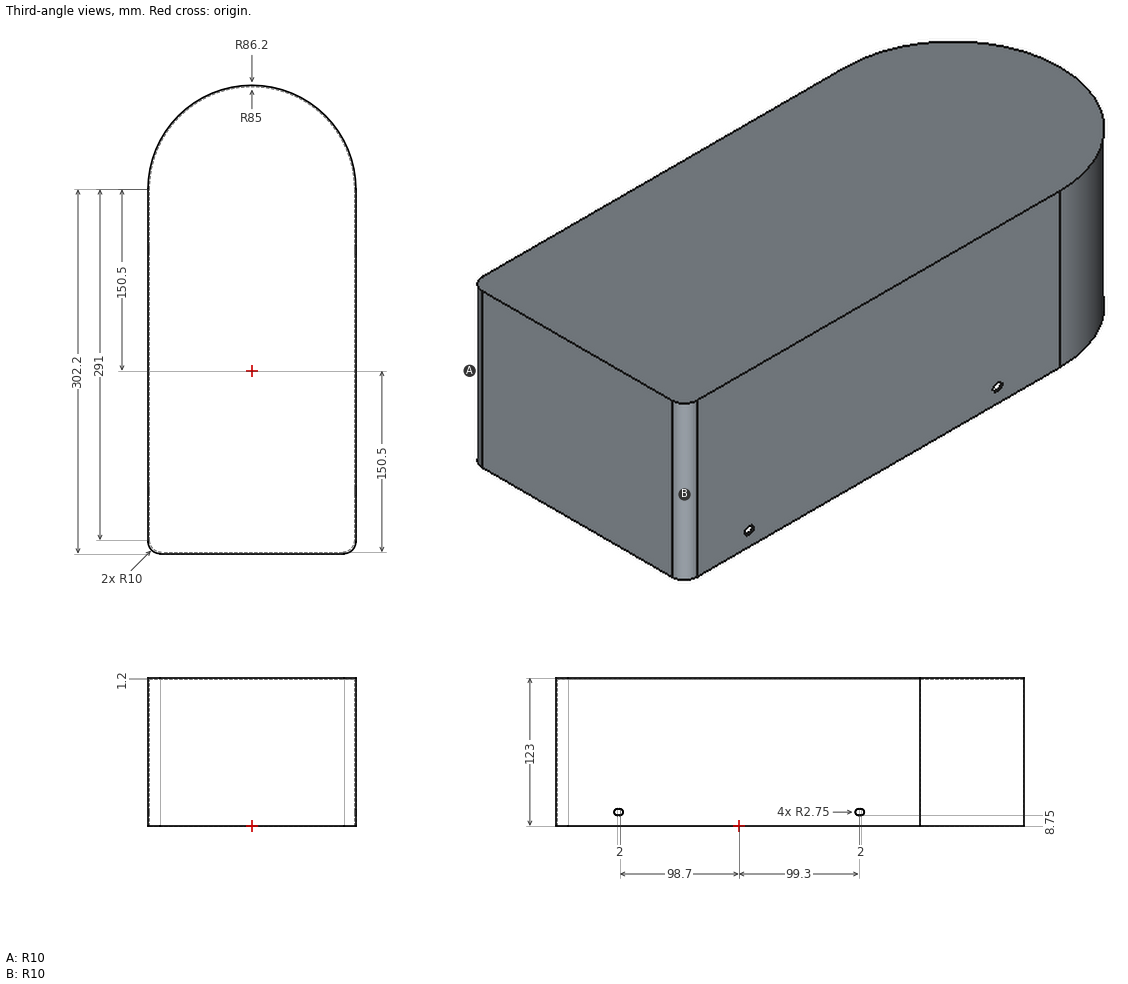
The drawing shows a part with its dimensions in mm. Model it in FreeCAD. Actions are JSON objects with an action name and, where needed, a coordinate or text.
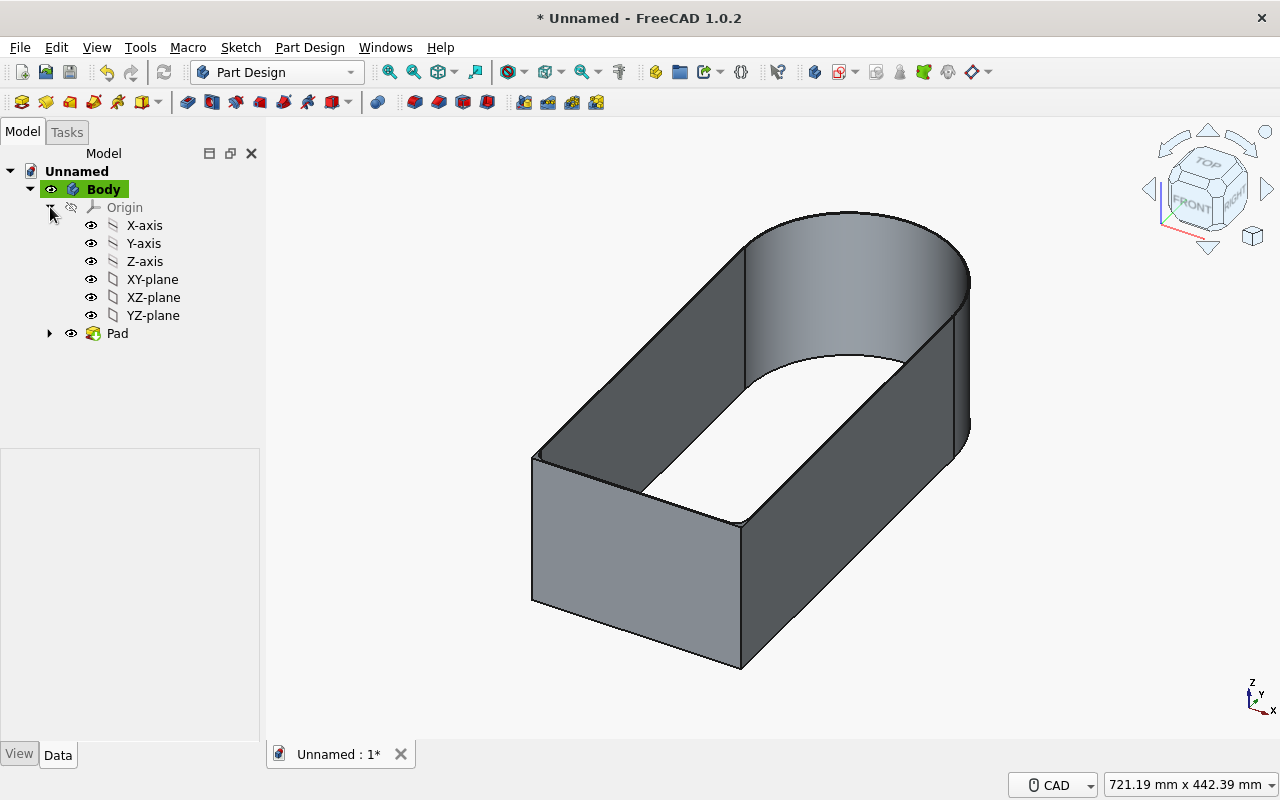
{"action": "left_click", "coordinate": [136, 279]}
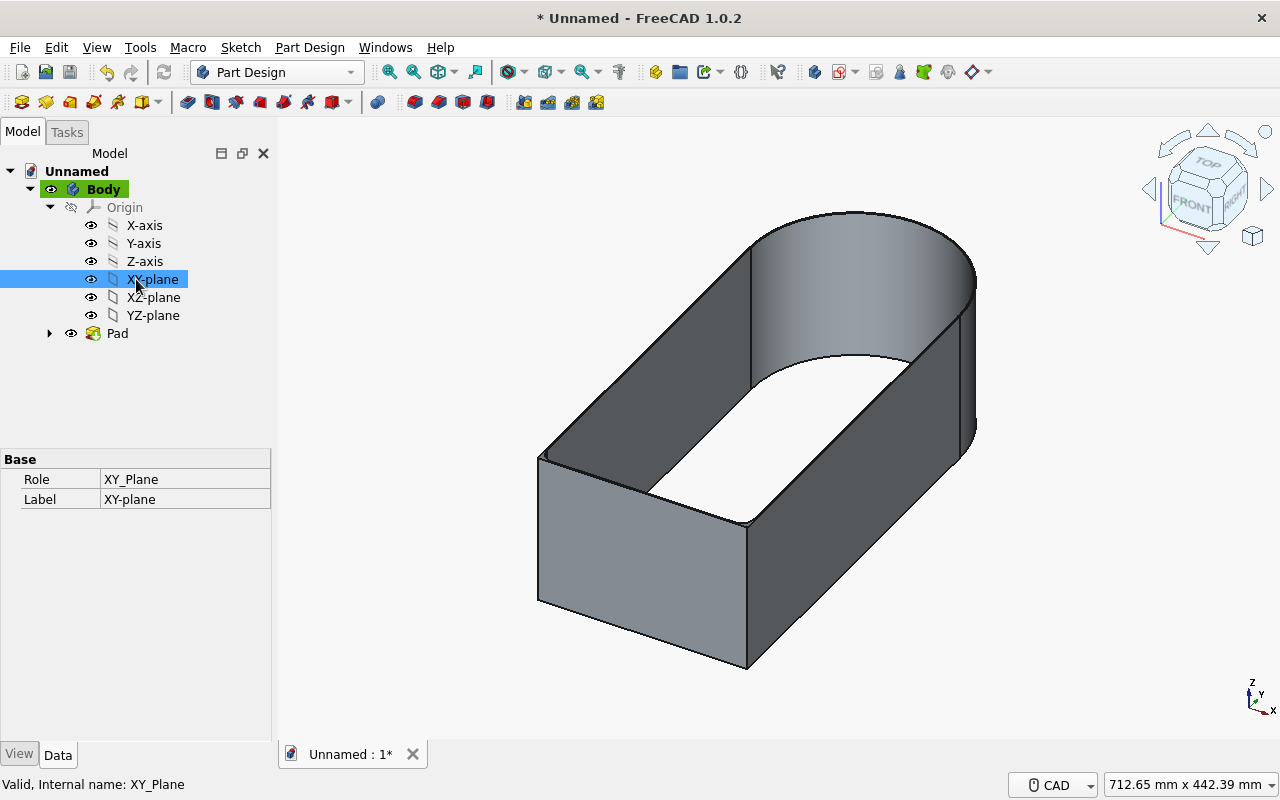
{"action": "left_click", "coordinate": [972, 72]}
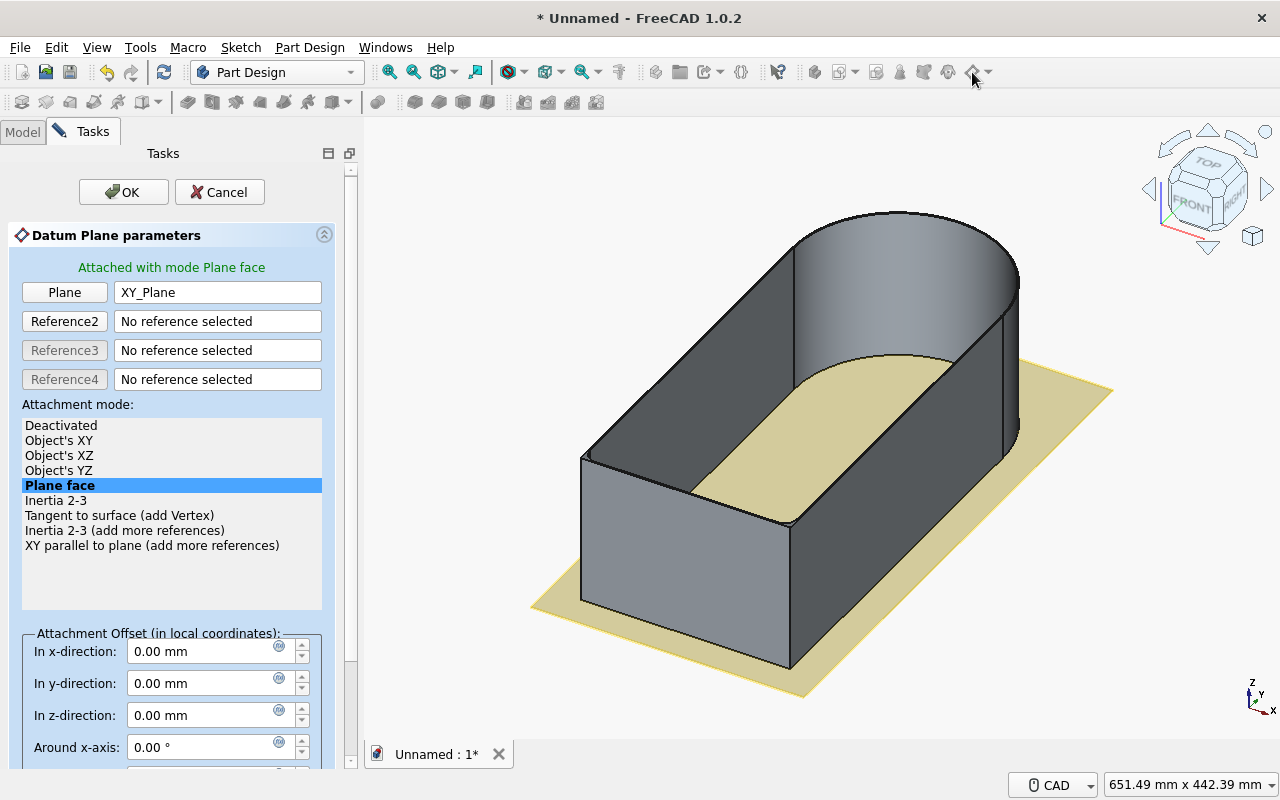
{"action": "triple_click", "coordinate": [210, 715]}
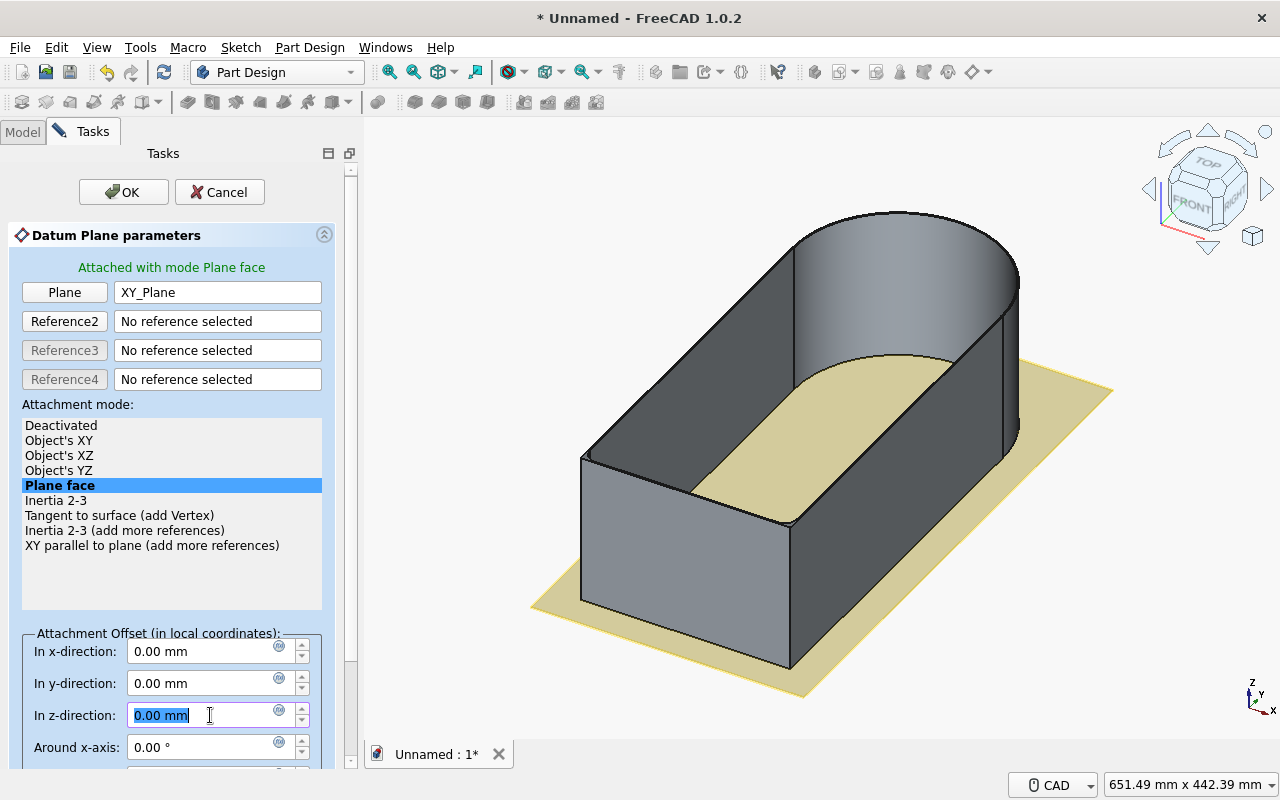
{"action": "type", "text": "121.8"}
{"action": "key", "text": "Tab"}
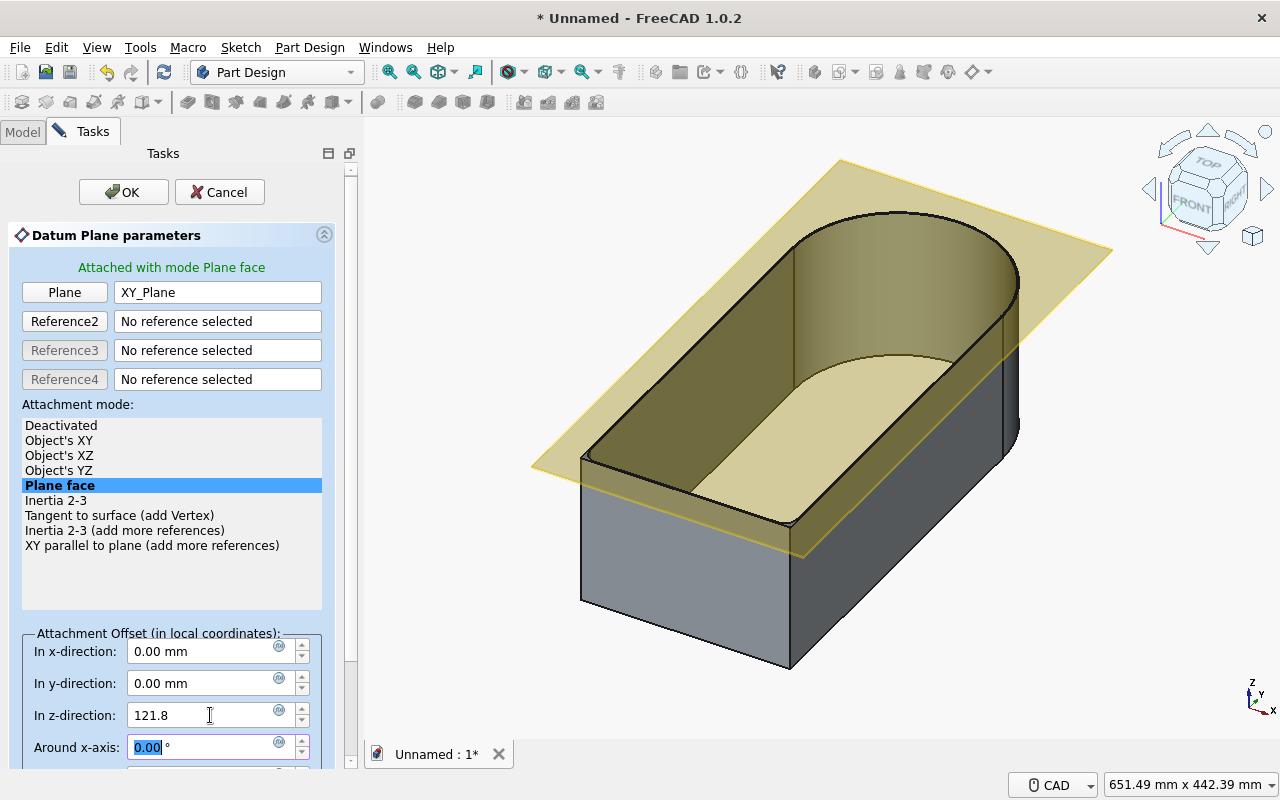
{"action": "left_click", "coordinate": [124, 192]}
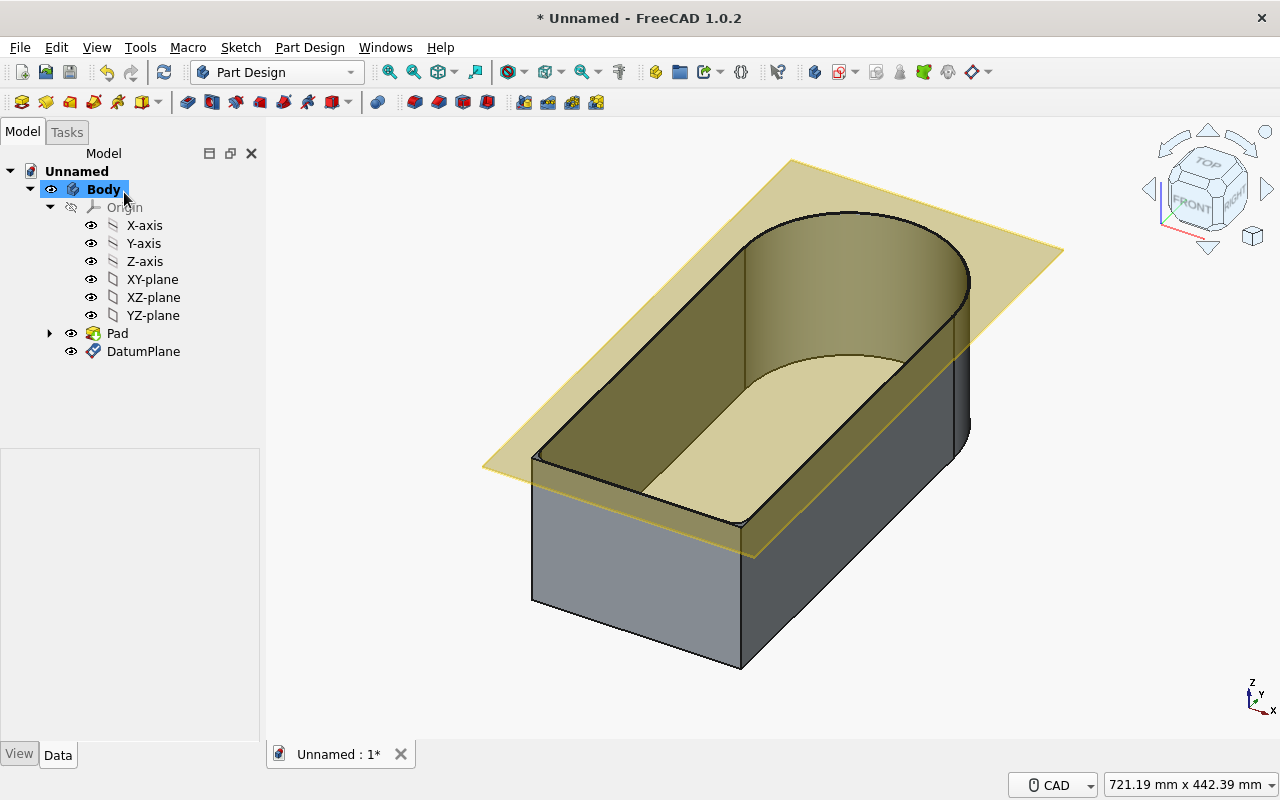
{"action": "left_click", "coordinate": [116, 351]}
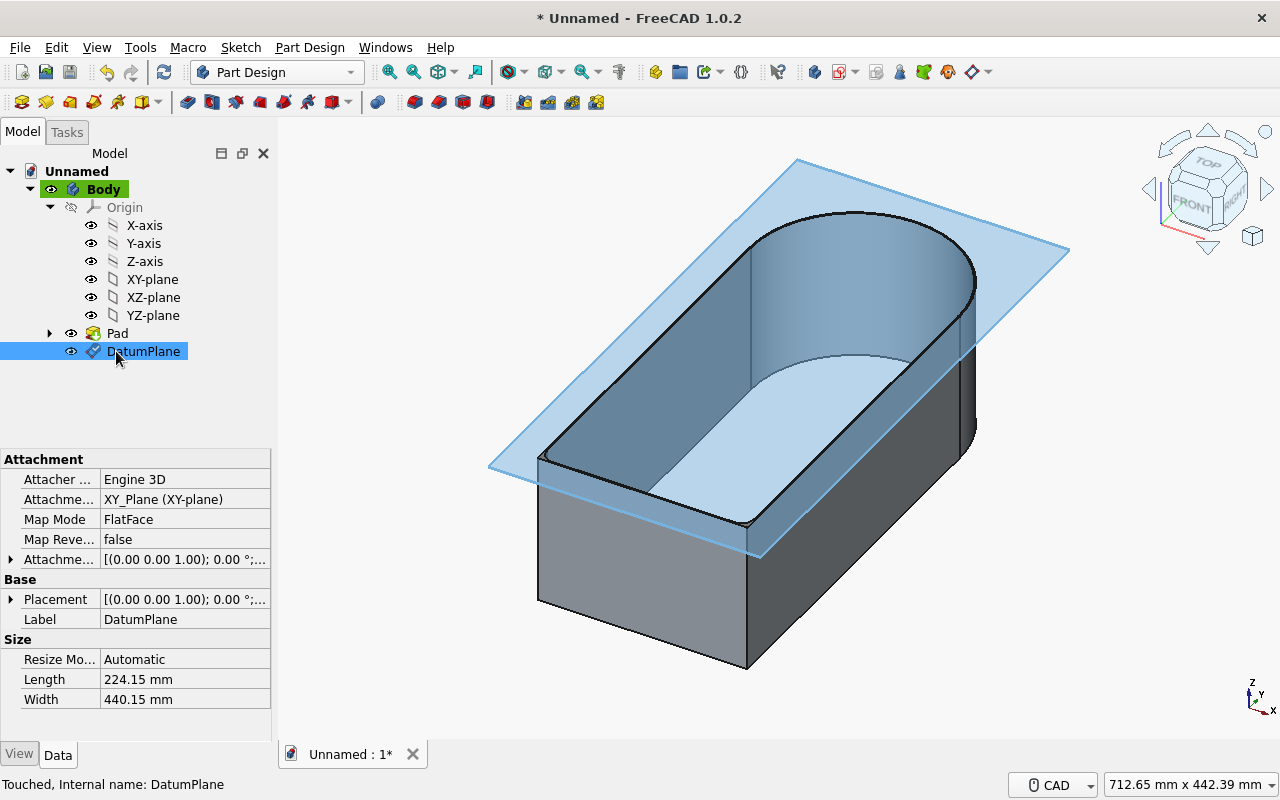
{"action": "left_click", "coordinate": [840, 72]}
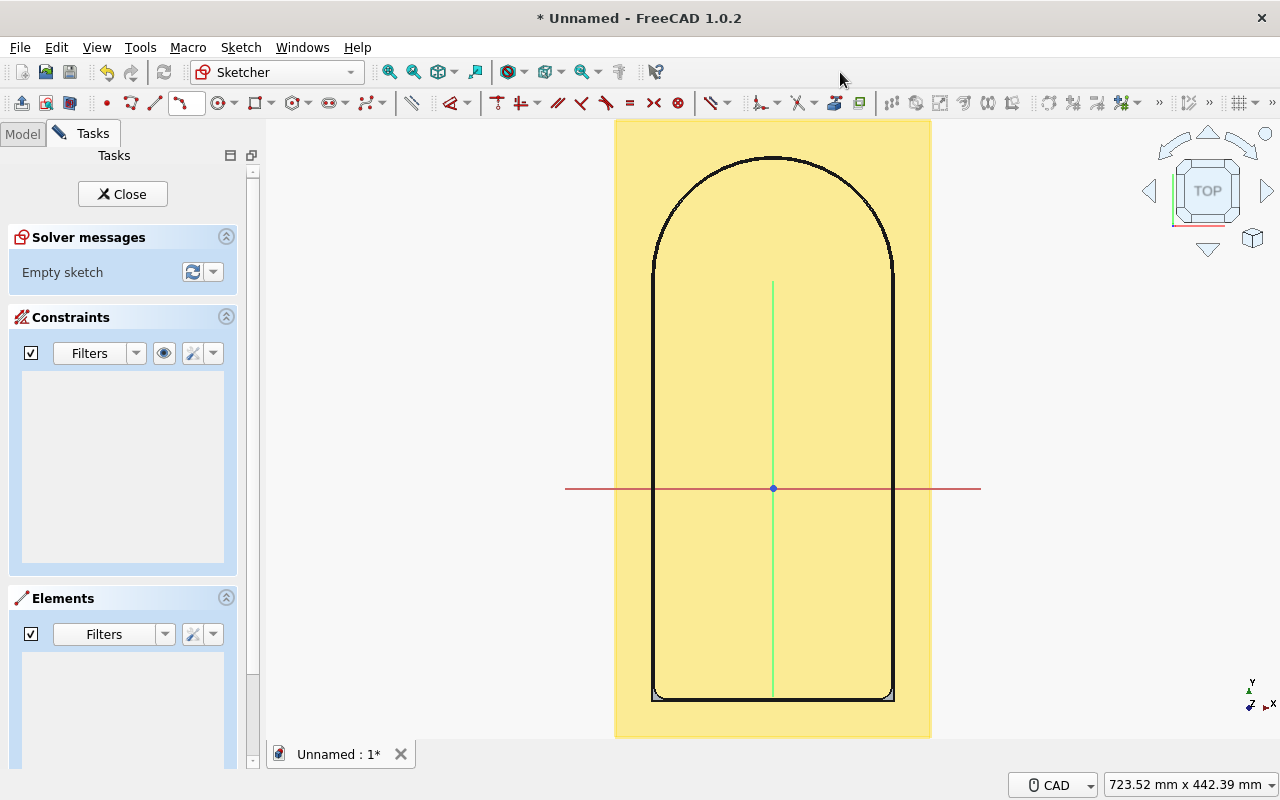
{"action": "key", "text": "q s"}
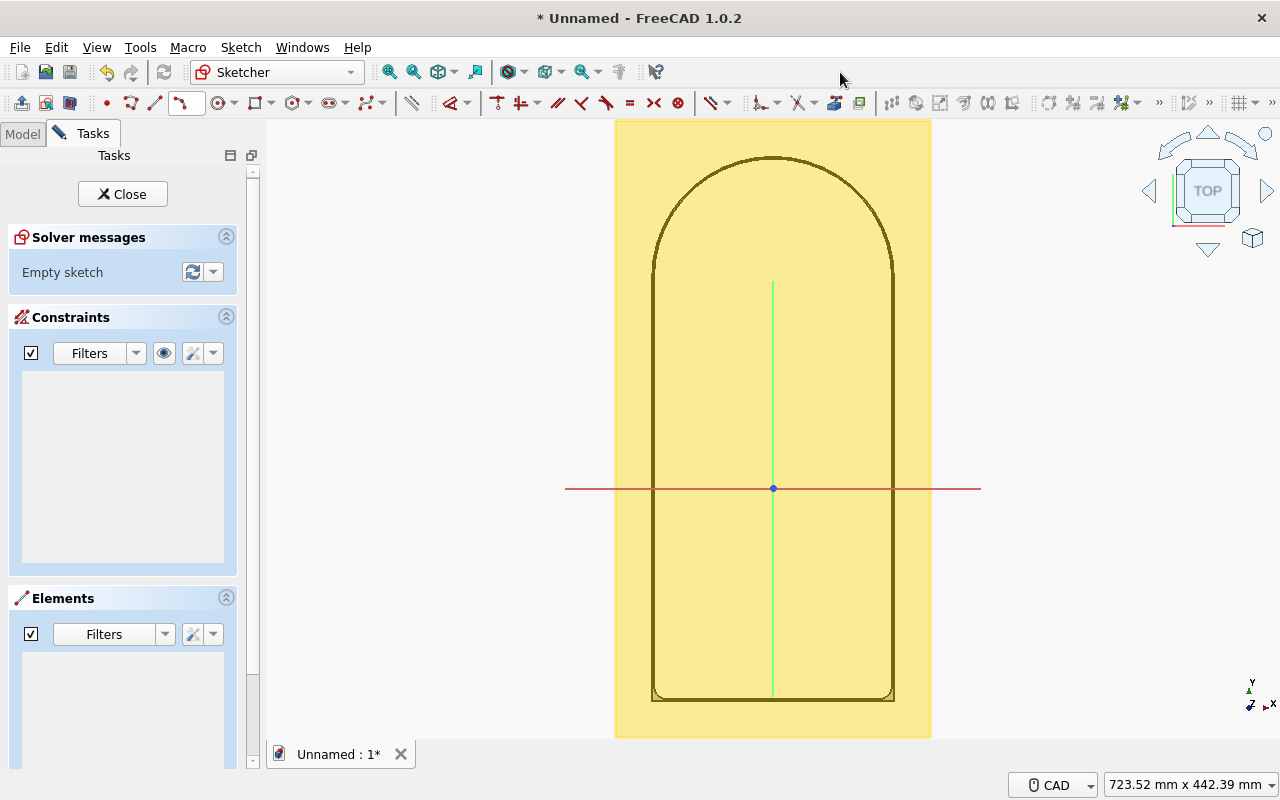
{"action": "scroll", "coordinate": [565, 429], "scroll_direction": "down", "scroll_amount": 2}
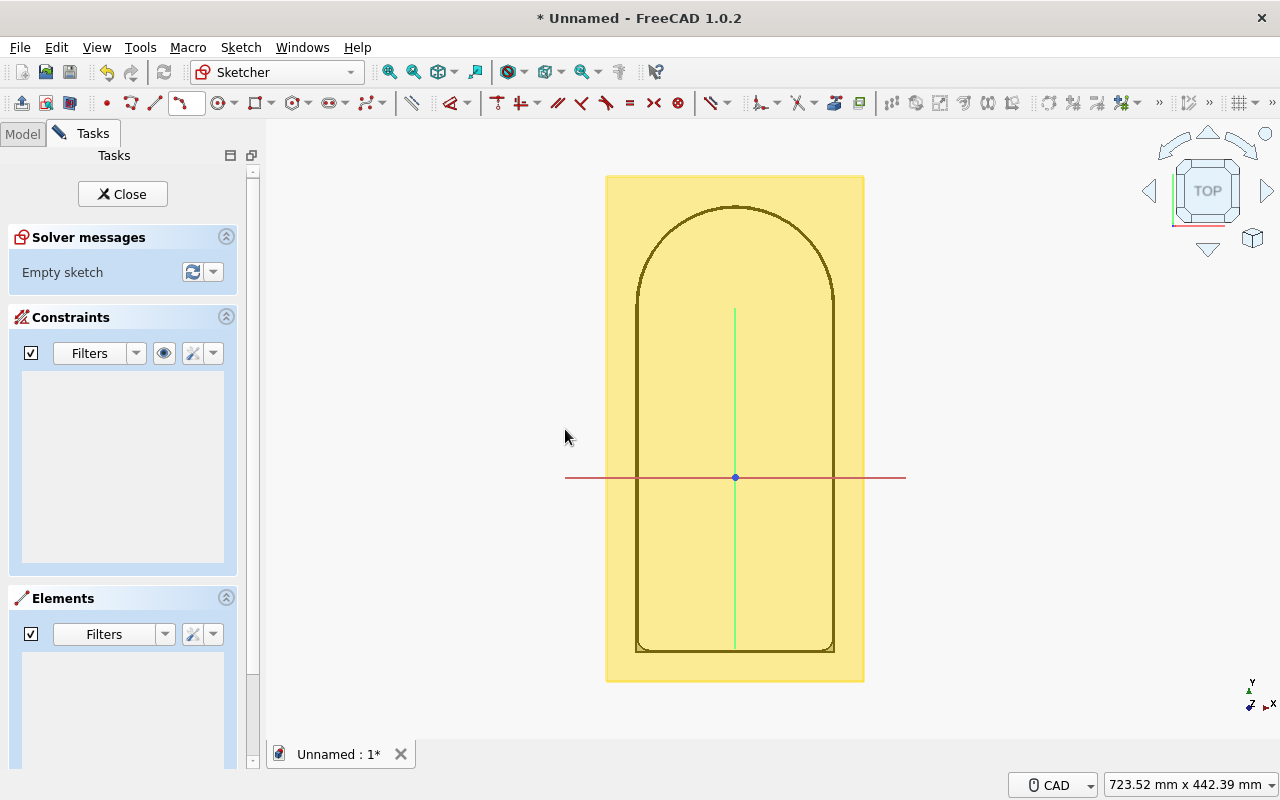
{"action": "left_click", "coordinate": [132, 104]}